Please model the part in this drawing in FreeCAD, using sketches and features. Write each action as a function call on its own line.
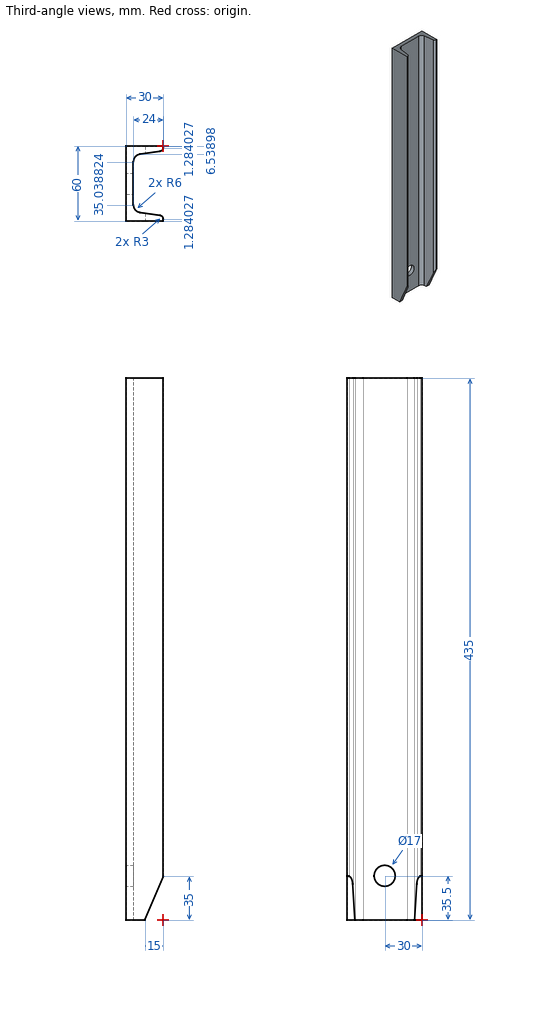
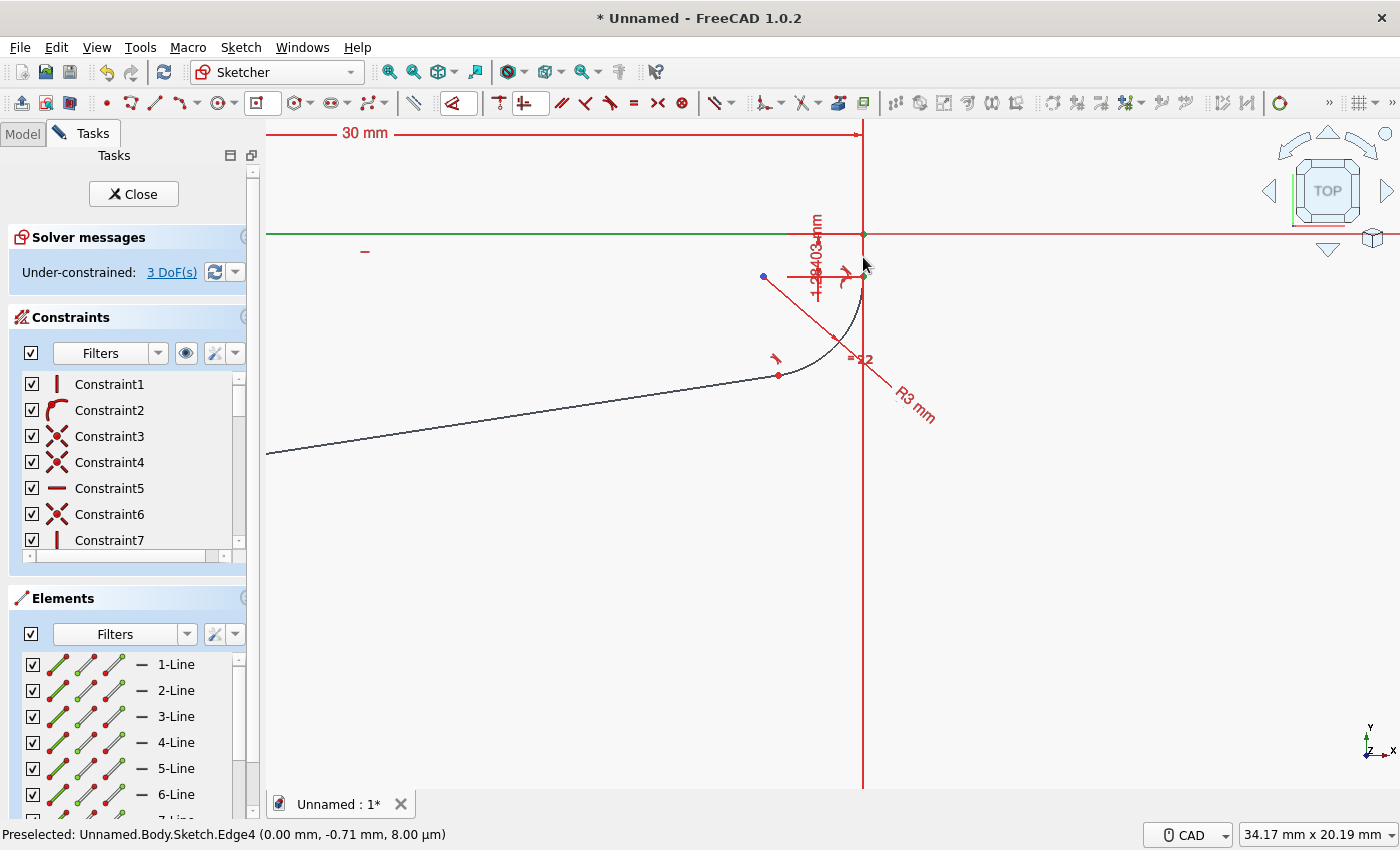
scroll(865, 258, down, 8)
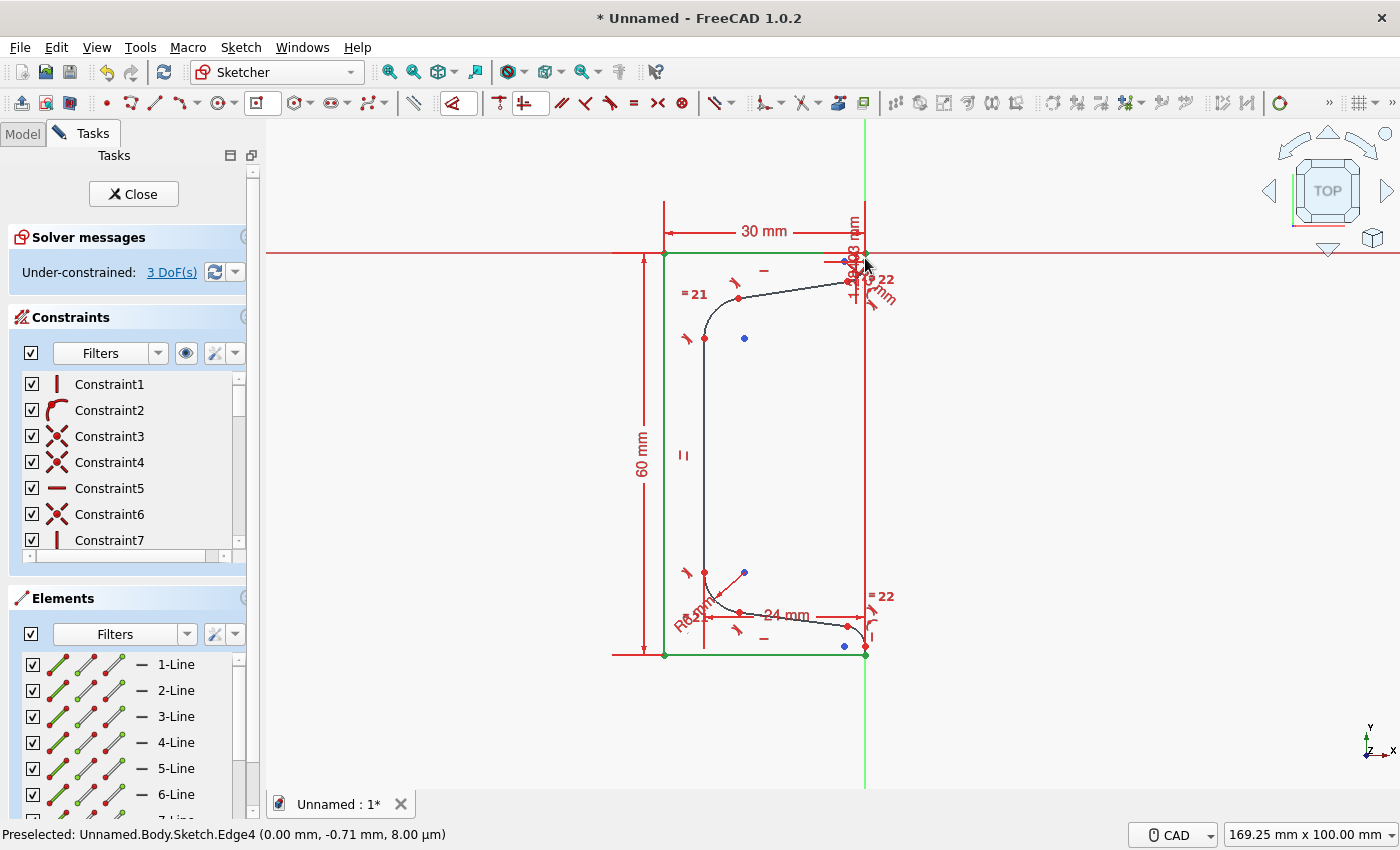
scroll(865, 653, up, 9)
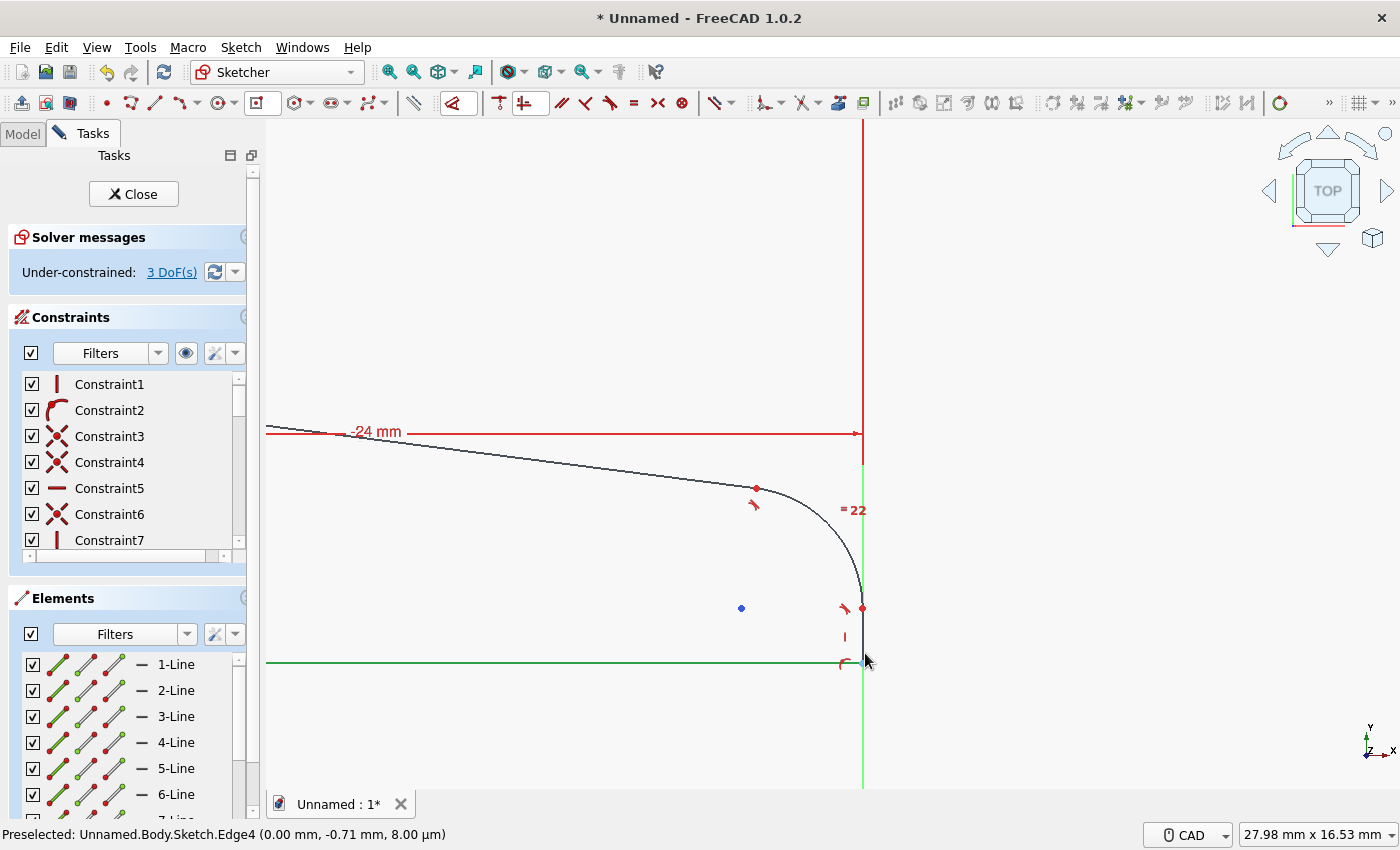
click(863, 647)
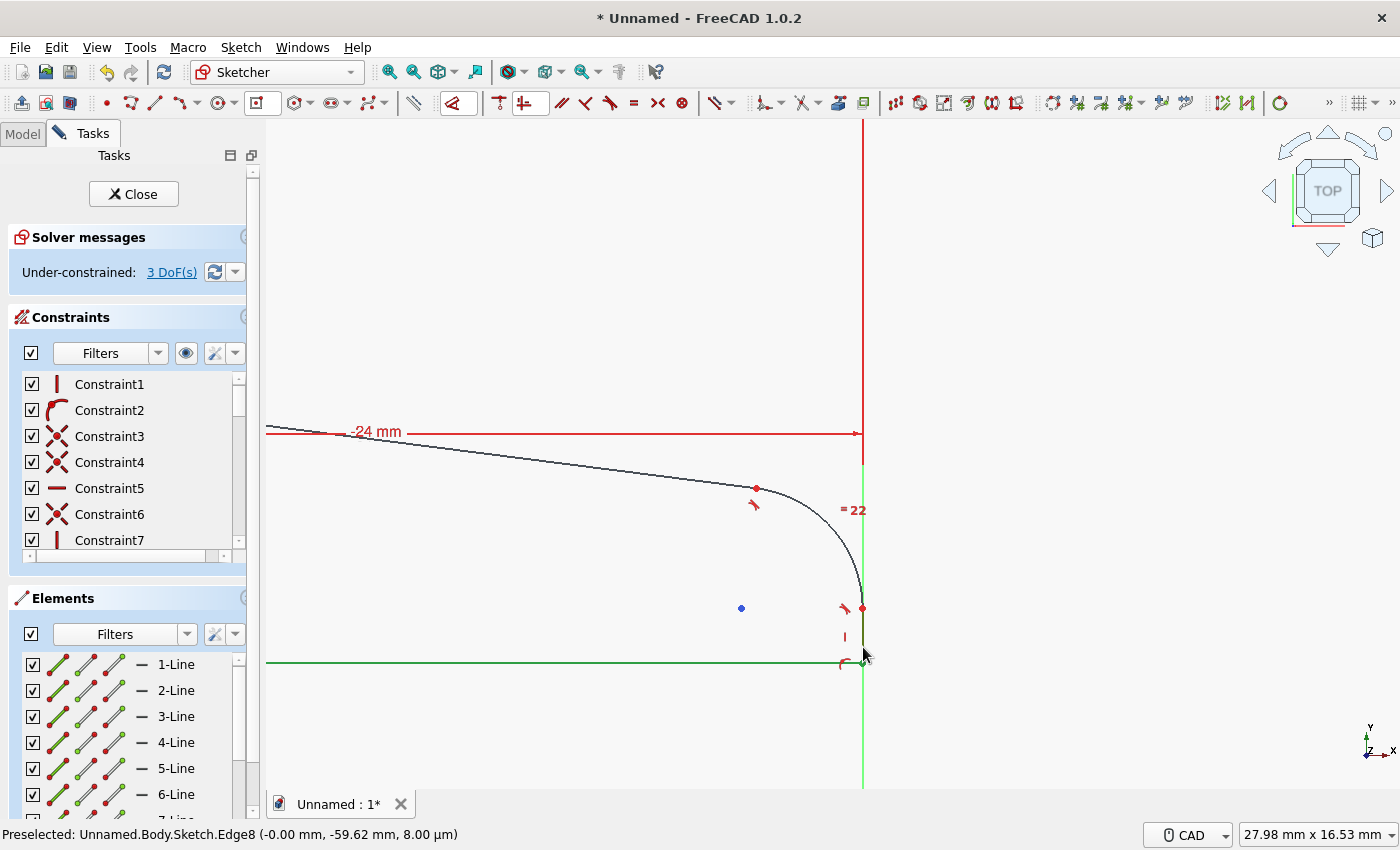
key(i)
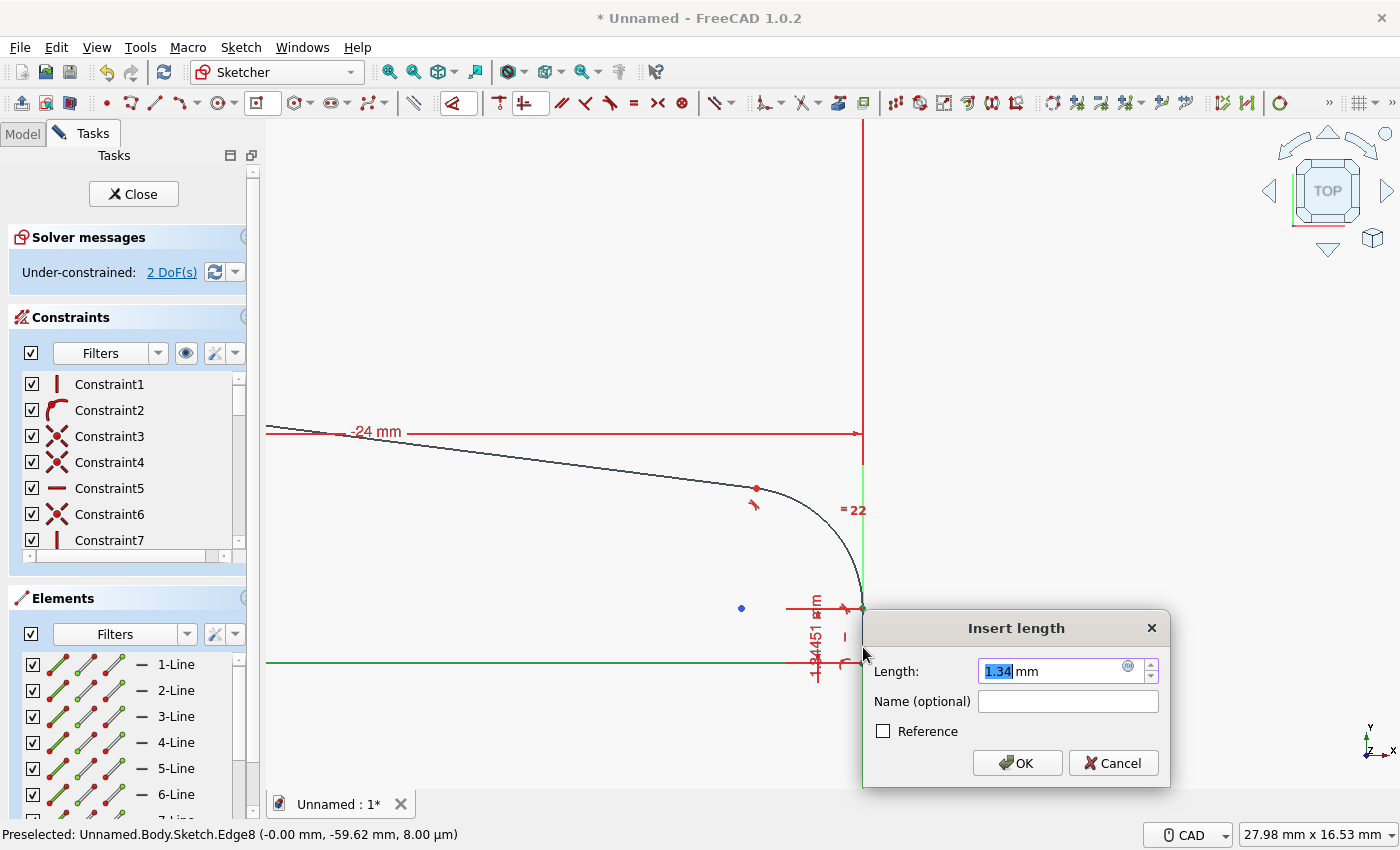
text(1.284027)
key(Return)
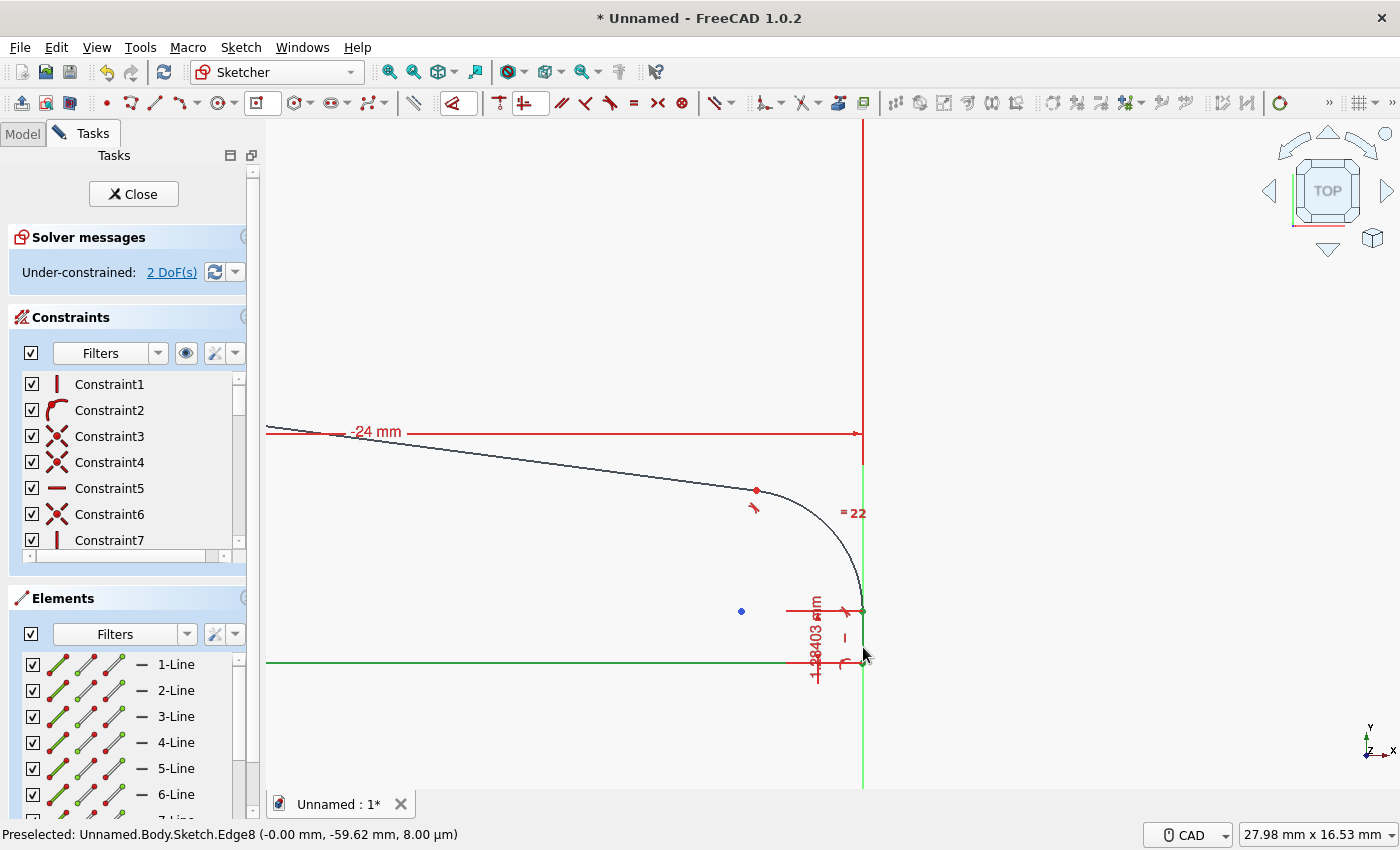
scroll(865, 653, down, 9)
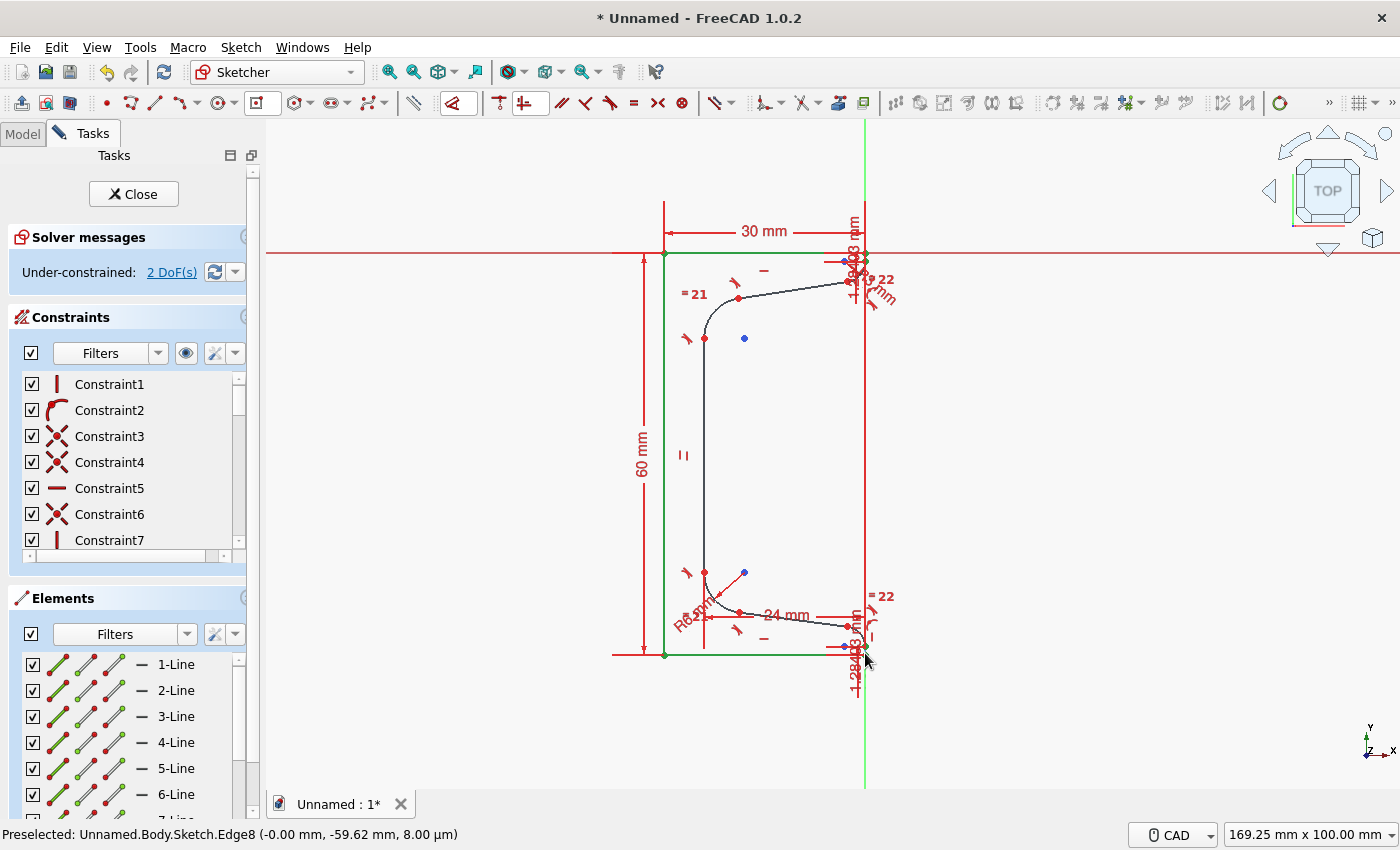
click(738, 299)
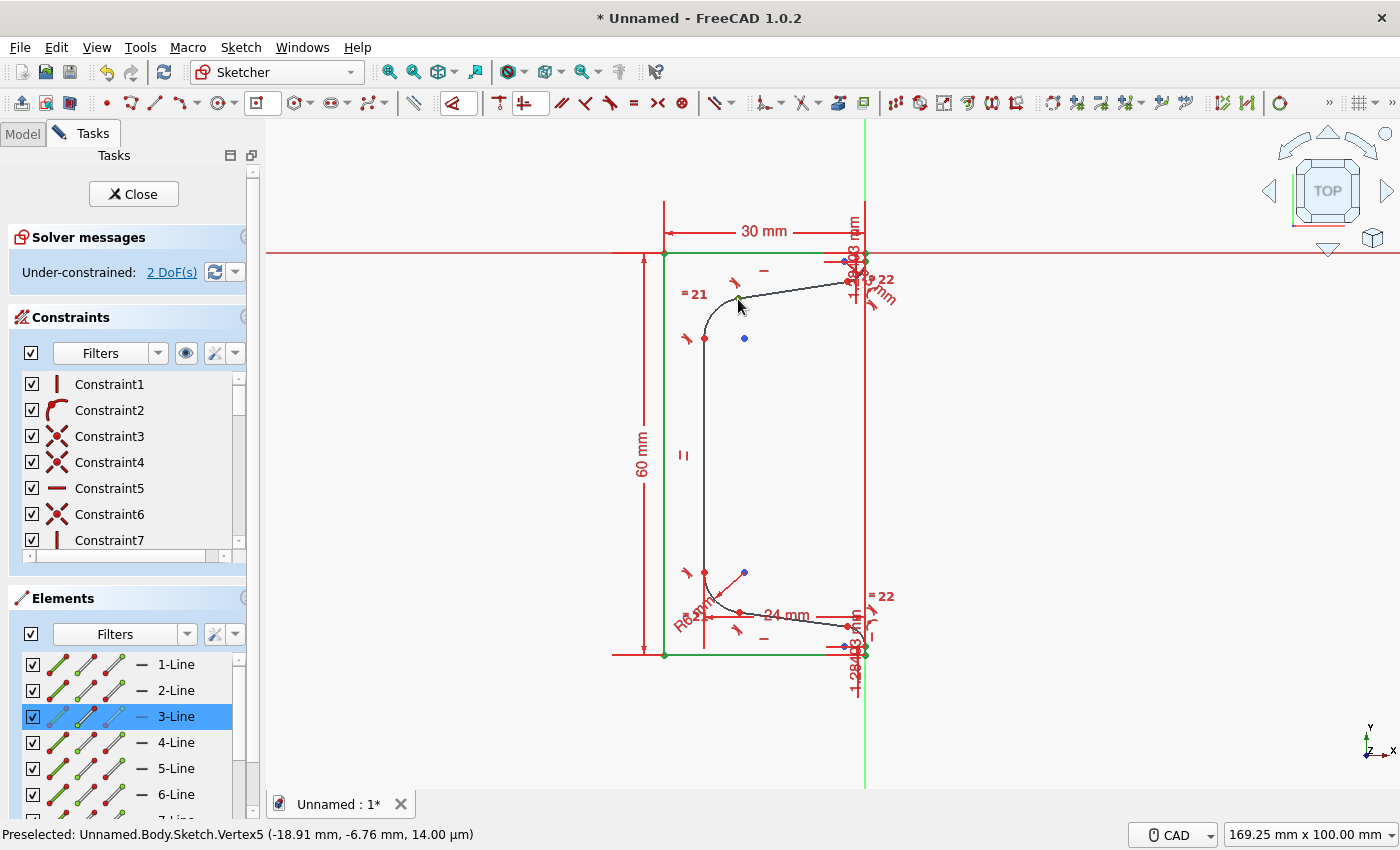
click(472, 104)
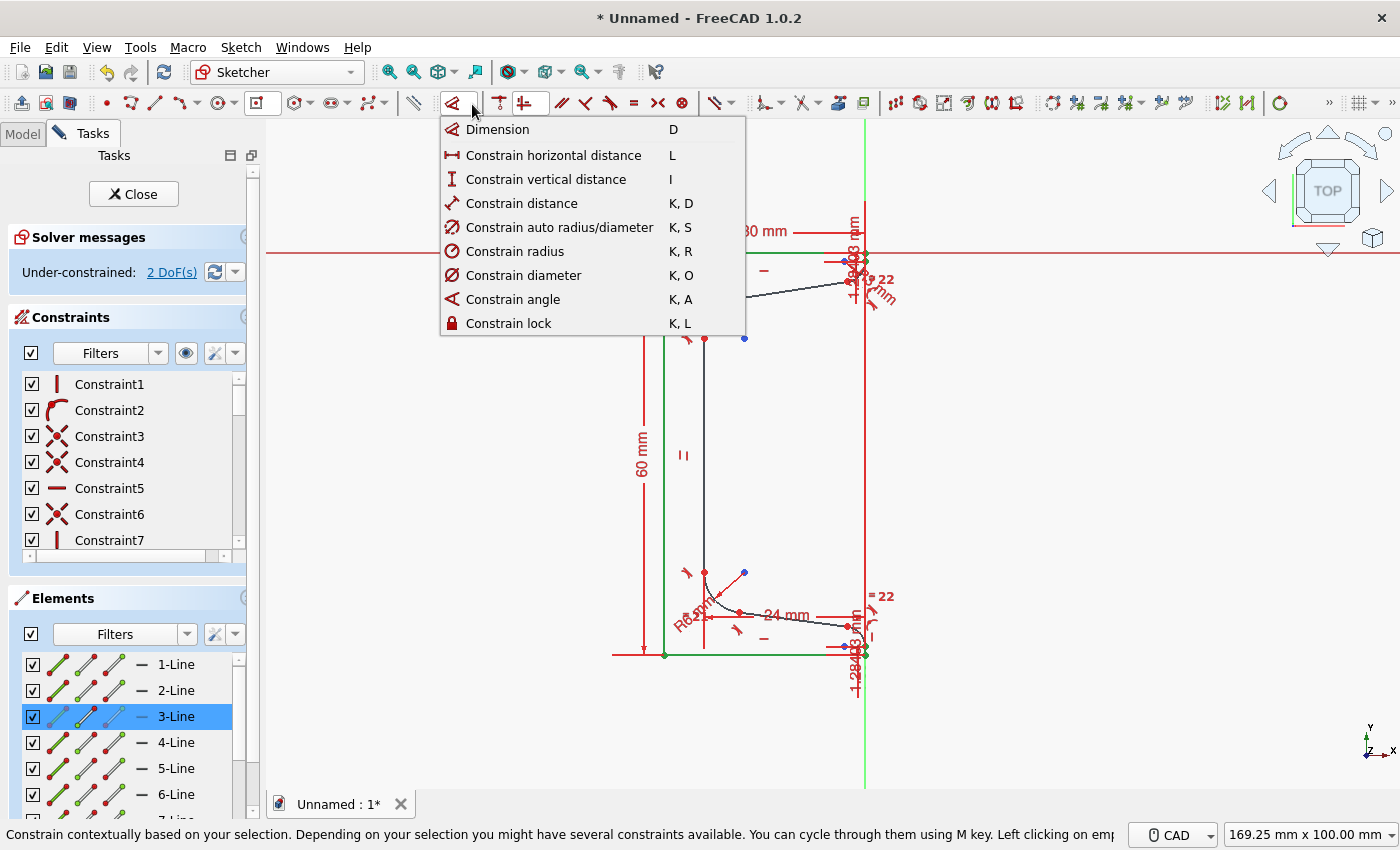
click(593, 179)